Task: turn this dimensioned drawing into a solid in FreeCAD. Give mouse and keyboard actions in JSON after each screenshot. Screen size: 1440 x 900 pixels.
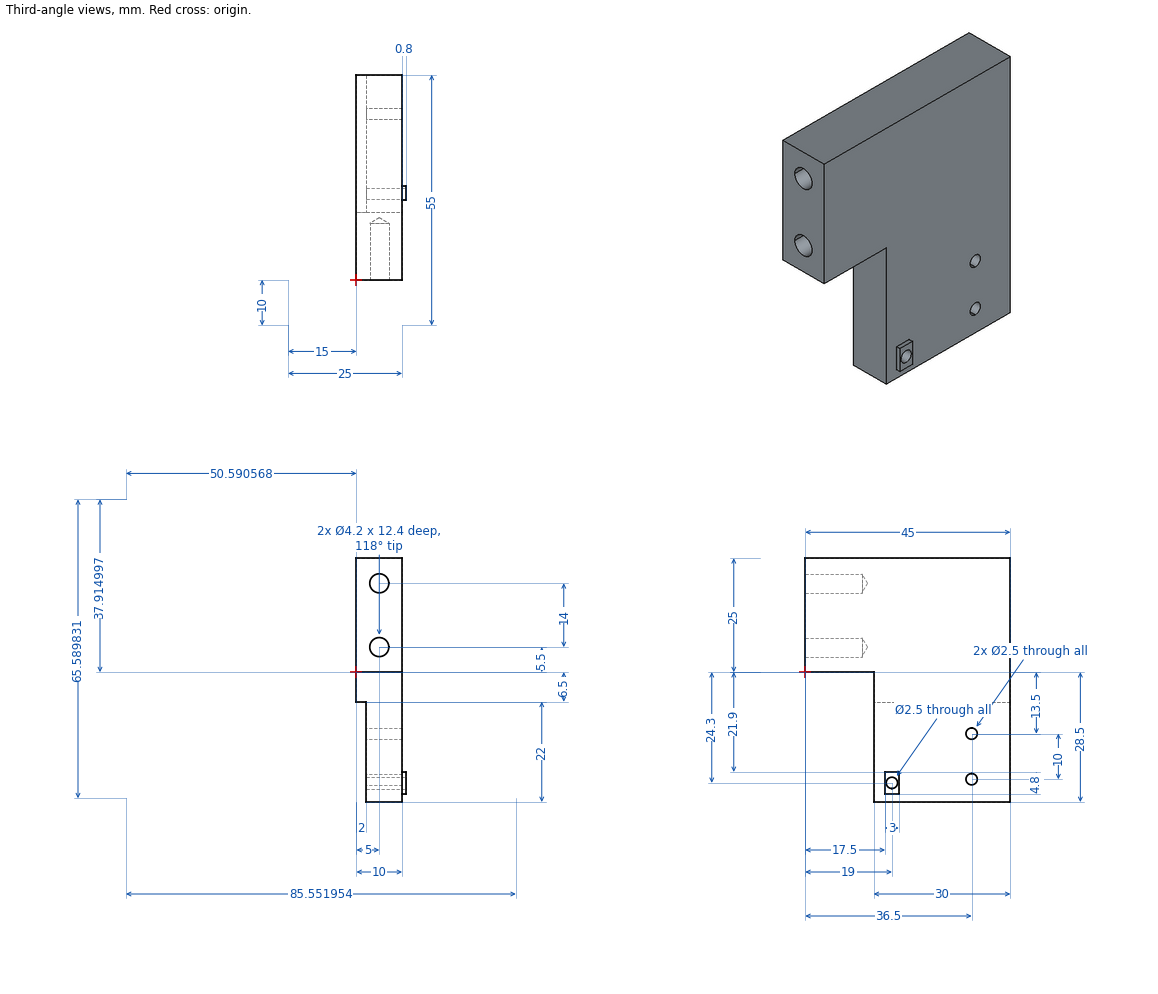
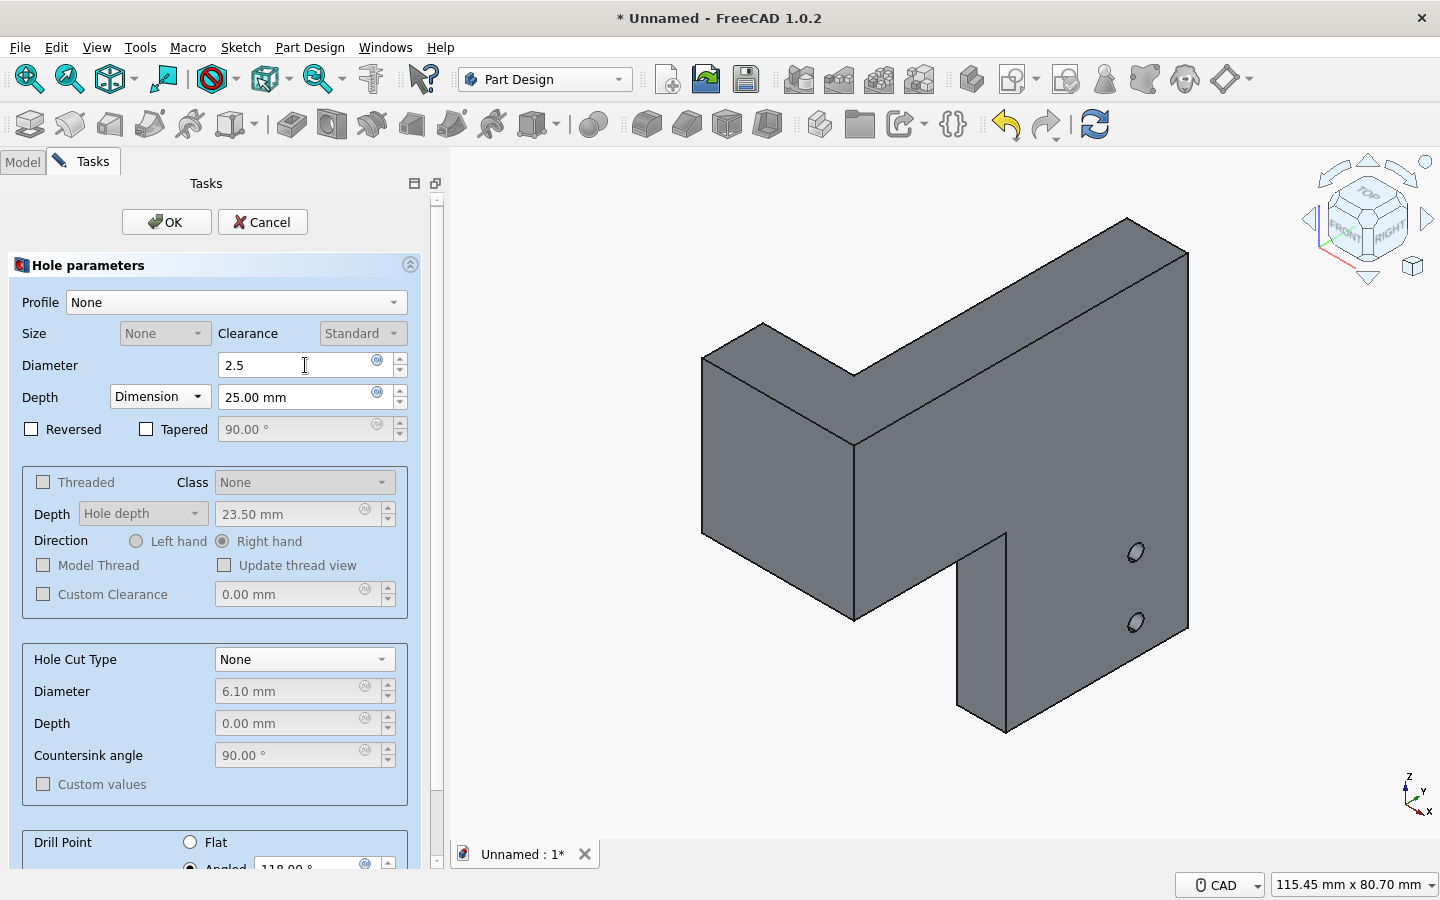
{"action": "left_click", "coordinate": [161, 396]}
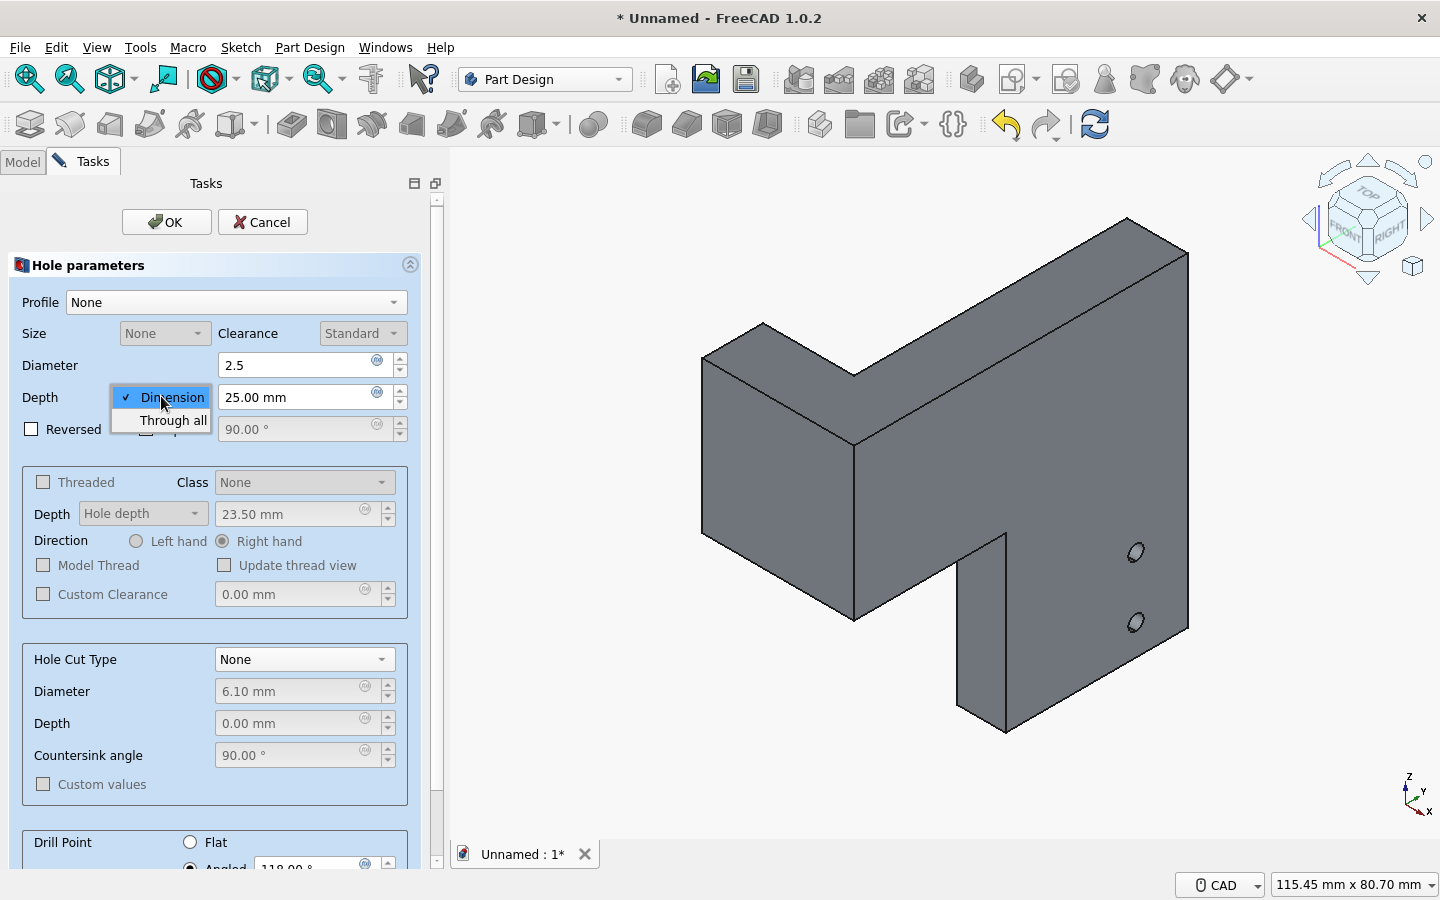
{"action": "left_click", "coordinate": [160, 420]}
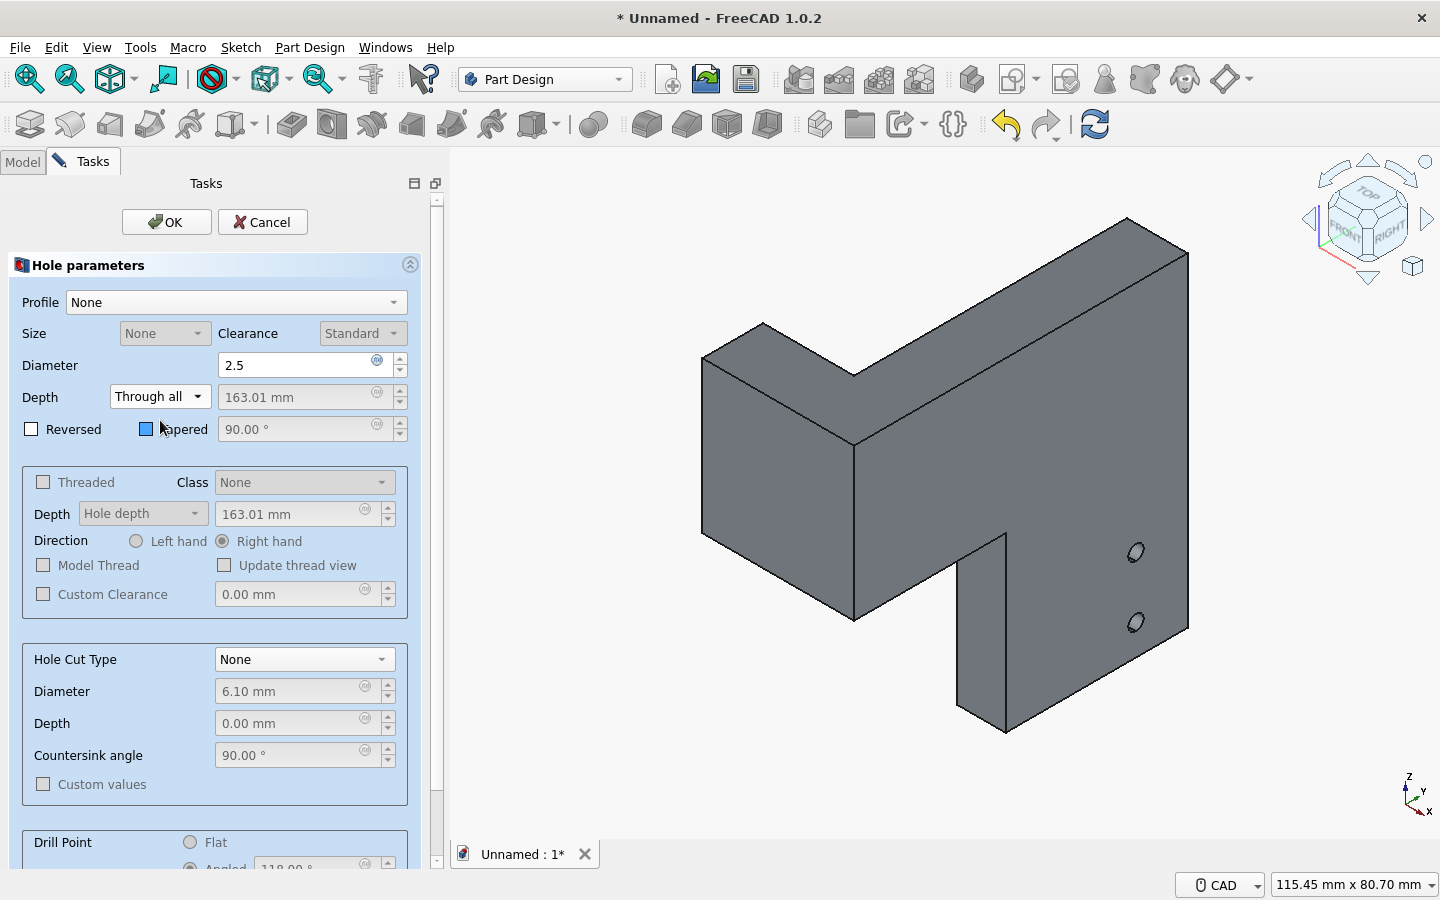
{"action": "left_click", "coordinate": [167, 222]}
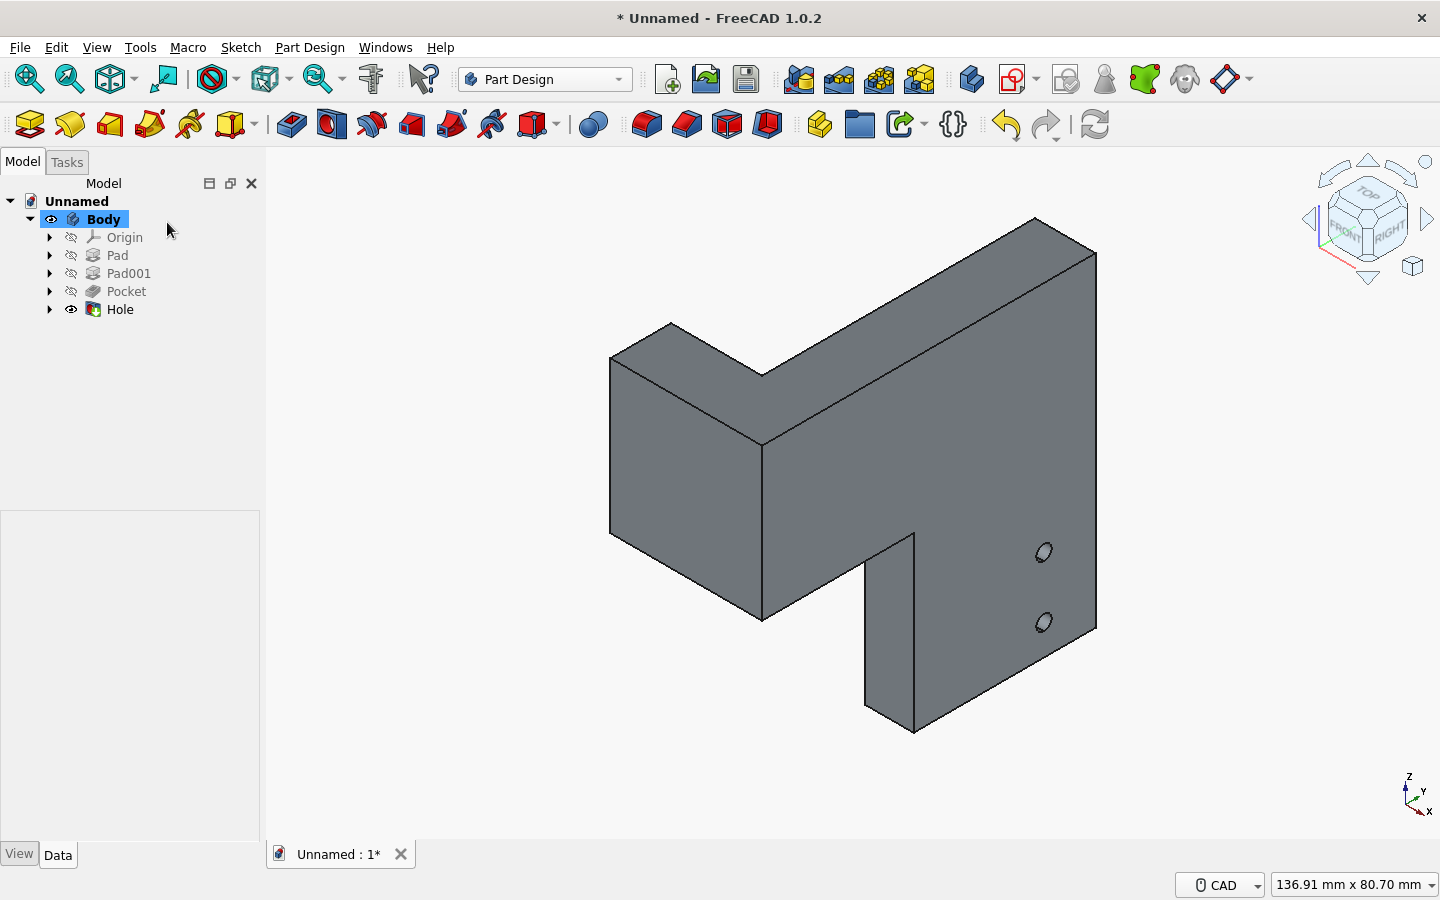
{"action": "left_click", "coordinate": [686, 488]}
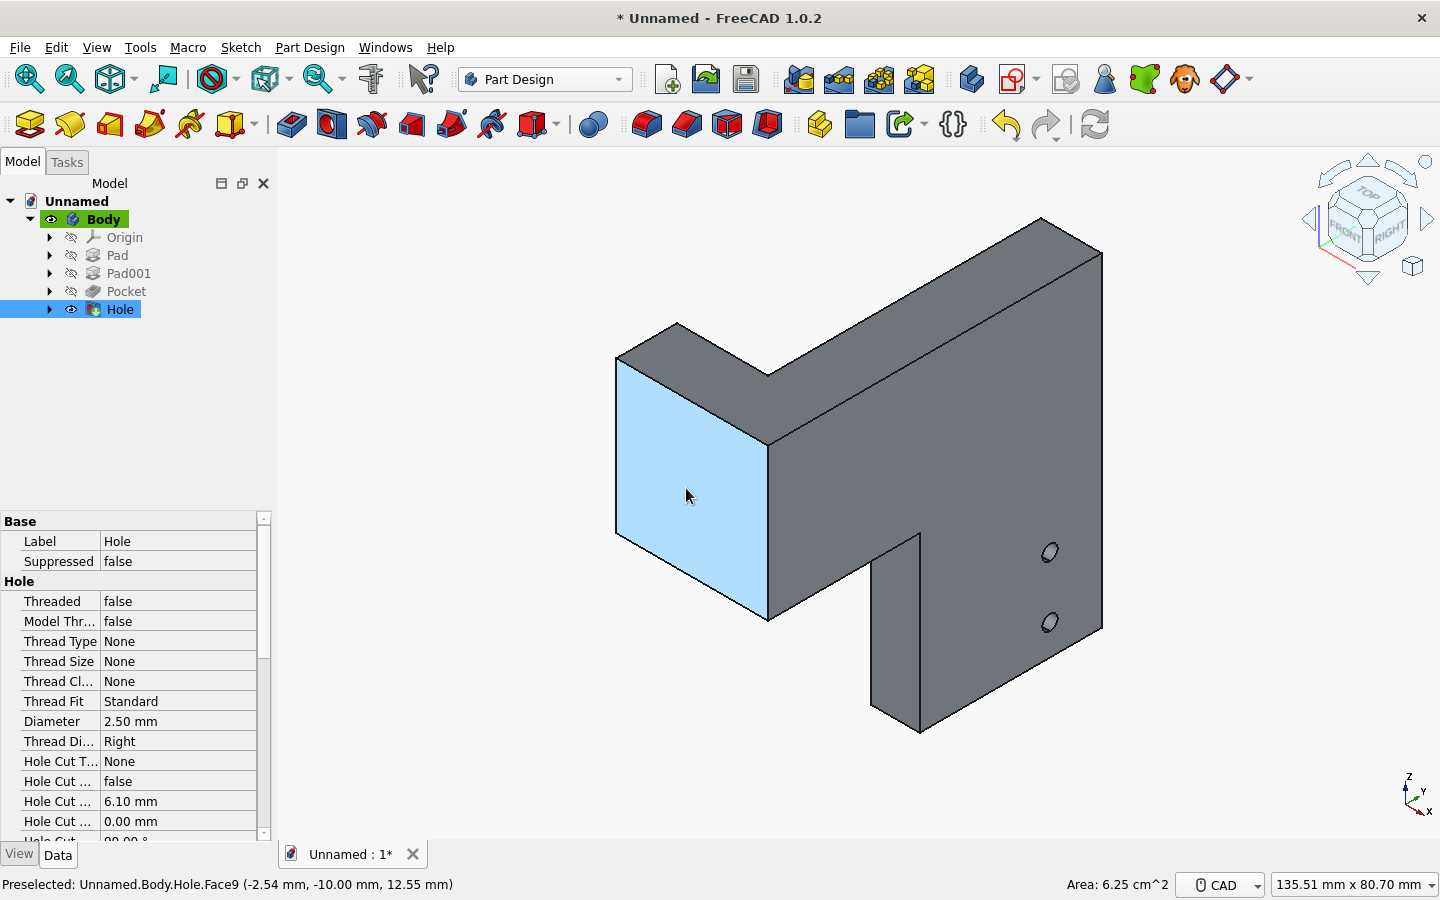
{"action": "left_click", "coordinate": [1012, 80]}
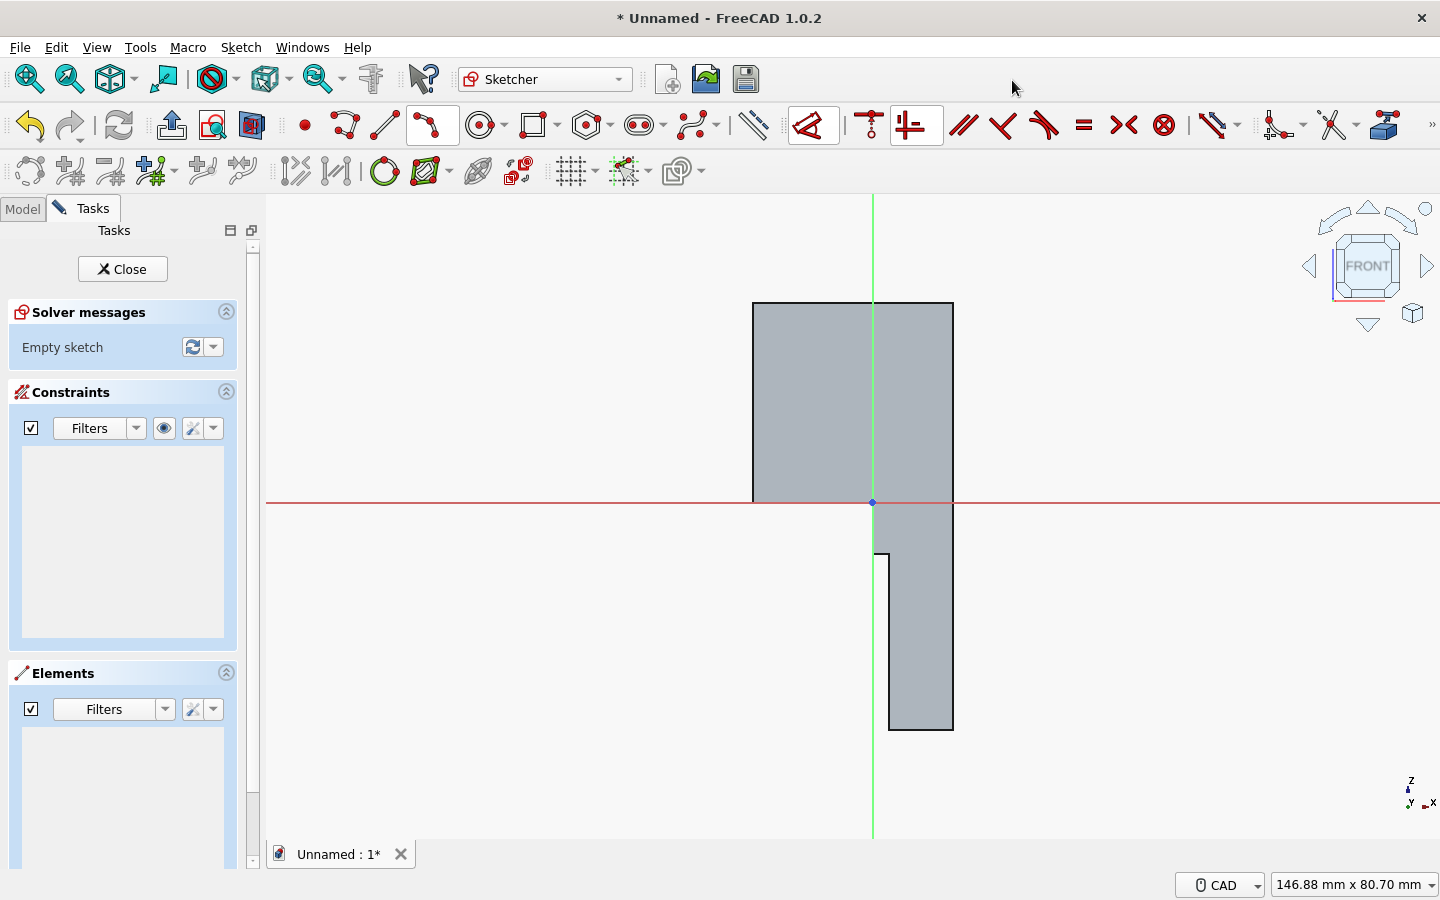
{"action": "scroll", "coordinate": [667, 765], "scroll_direction": "down", "scroll_amount": 1}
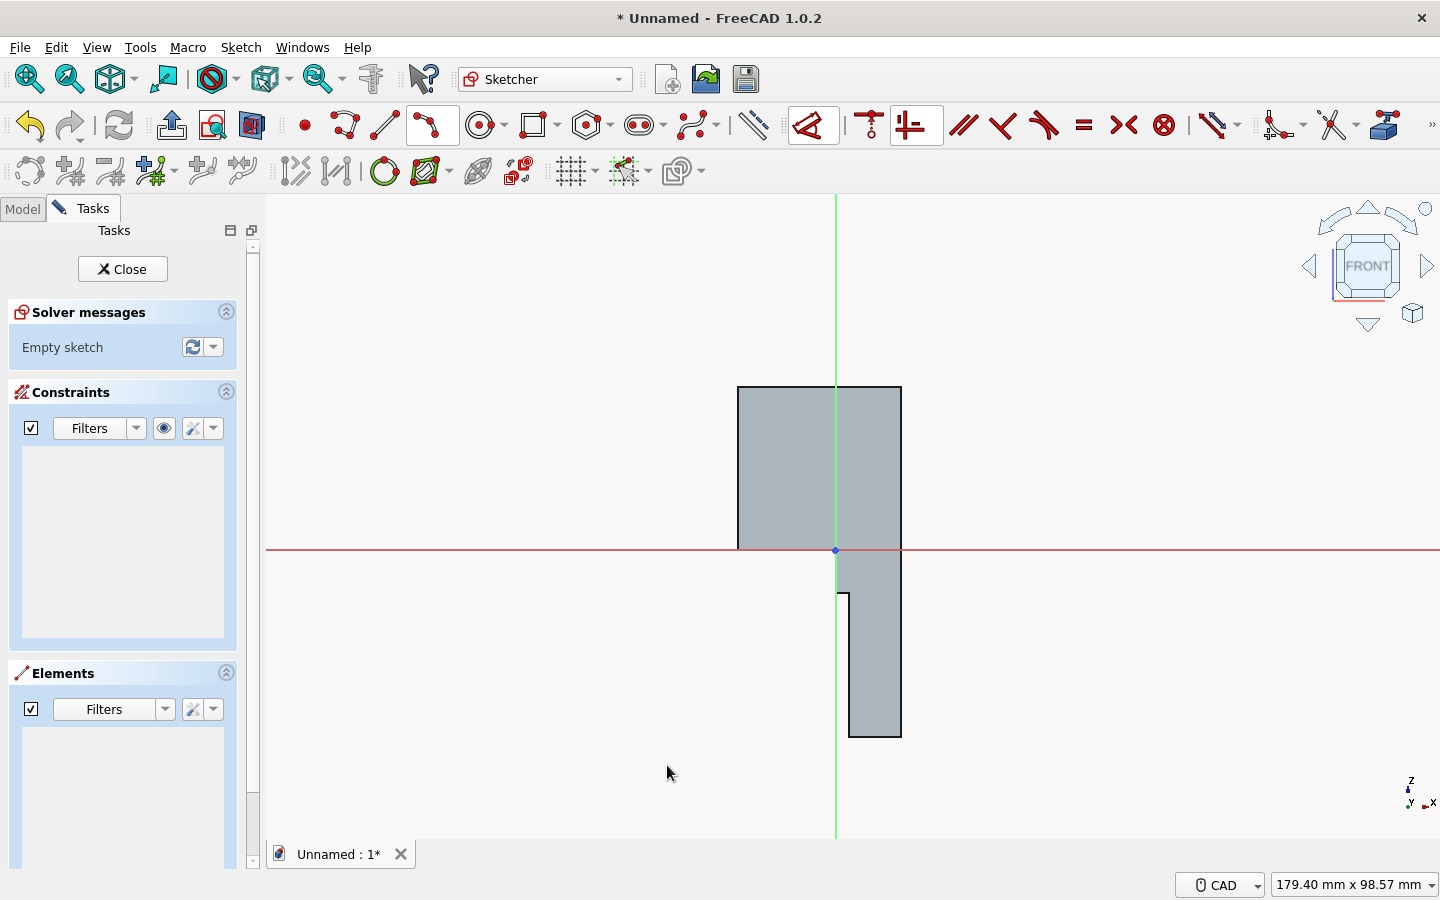
{"action": "left_click", "coordinate": [534, 126]}